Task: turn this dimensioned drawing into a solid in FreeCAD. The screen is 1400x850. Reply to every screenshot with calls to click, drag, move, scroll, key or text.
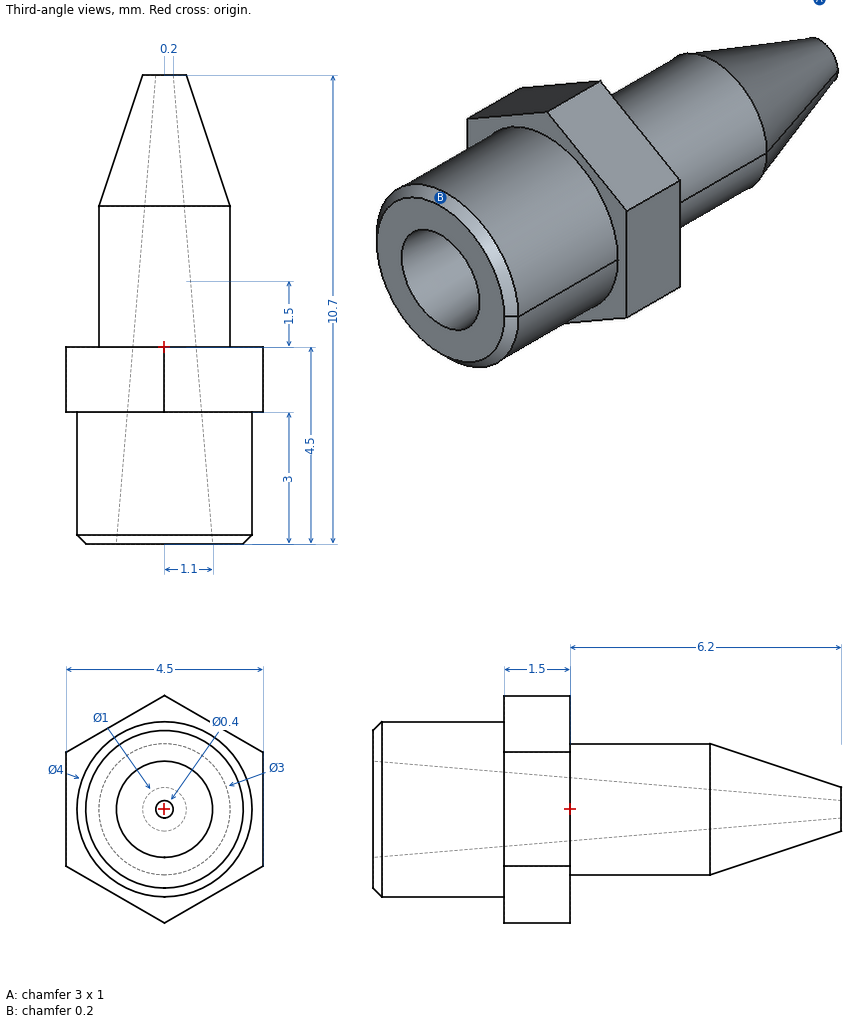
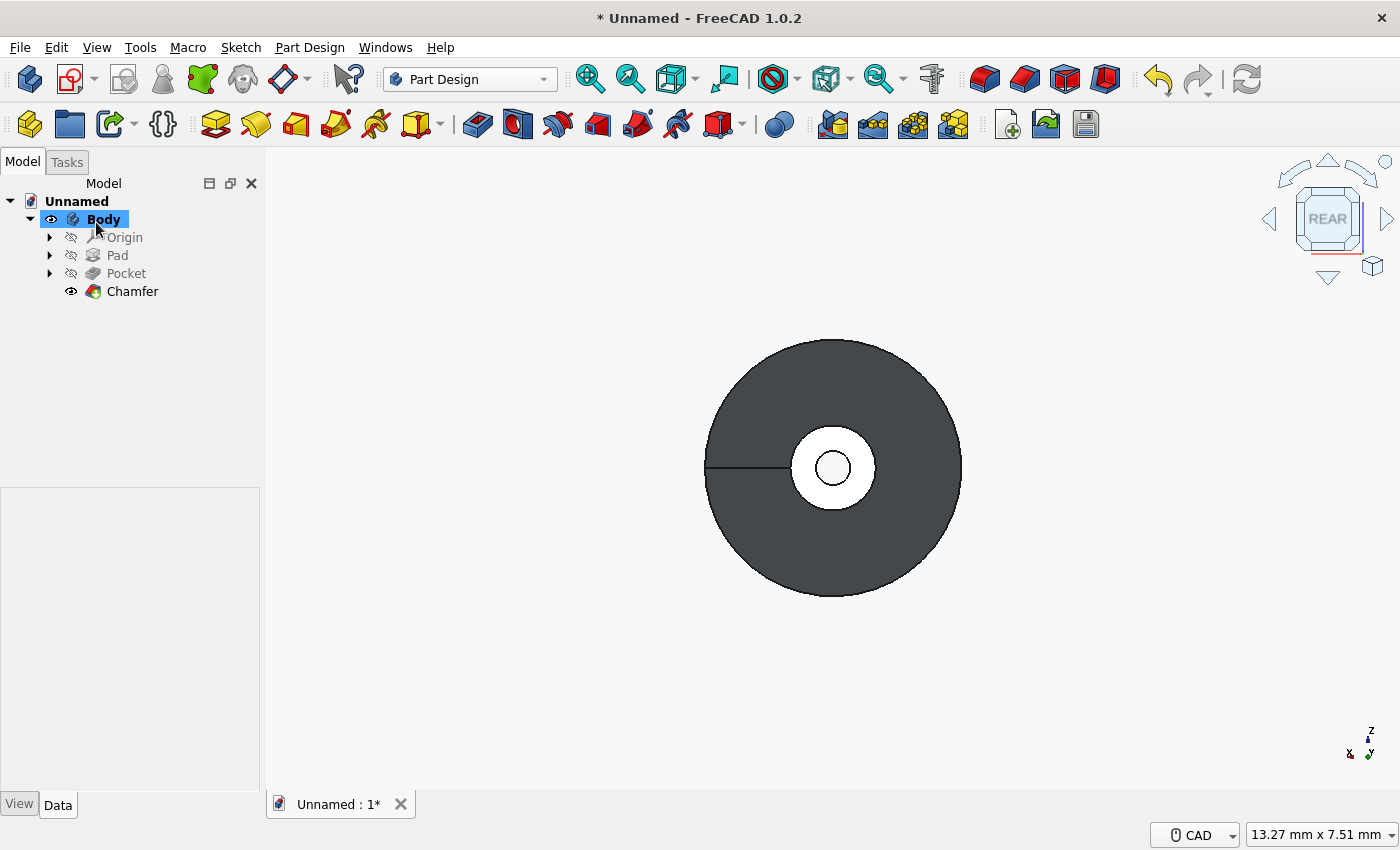
click(592, 80)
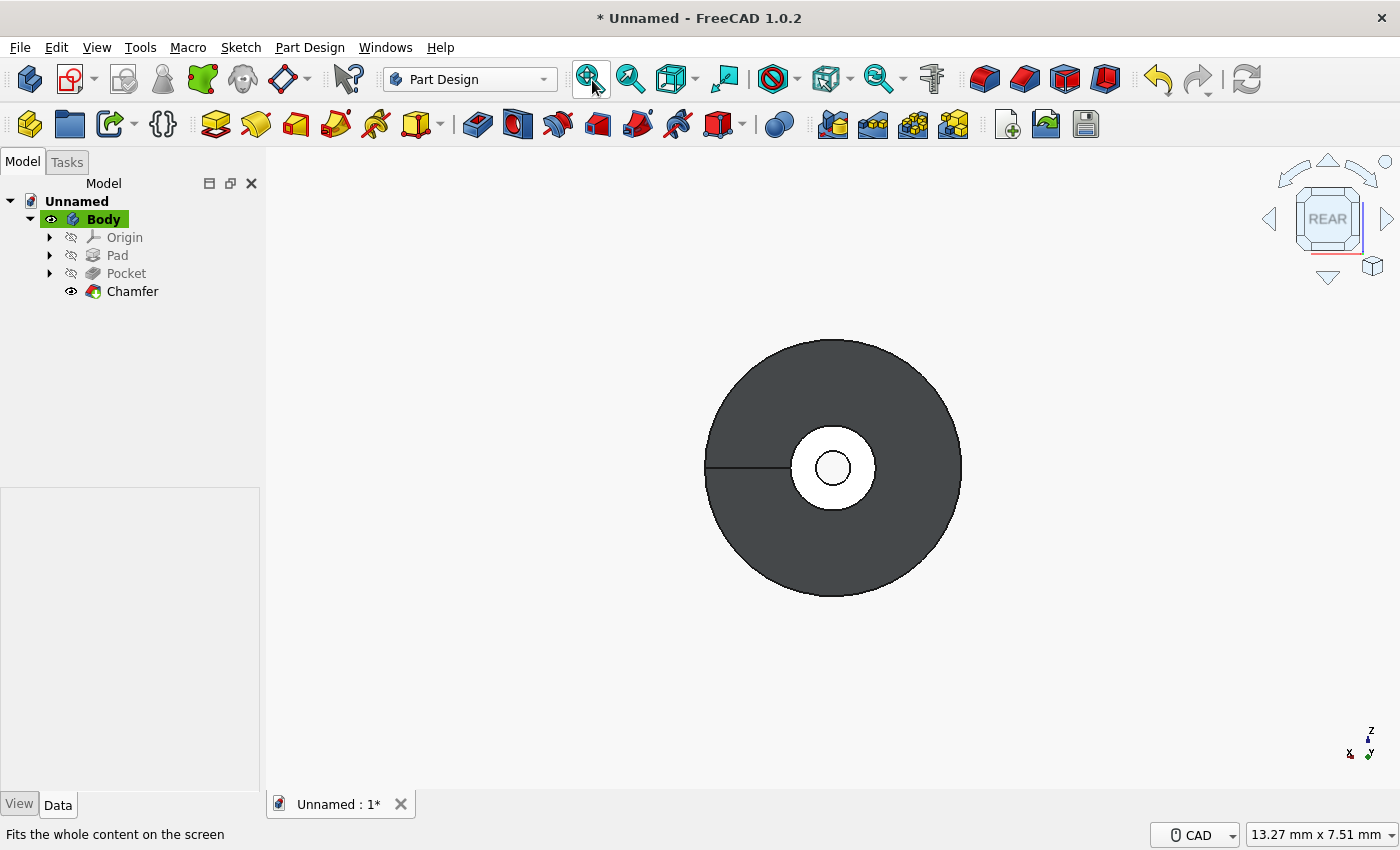
click(70, 80)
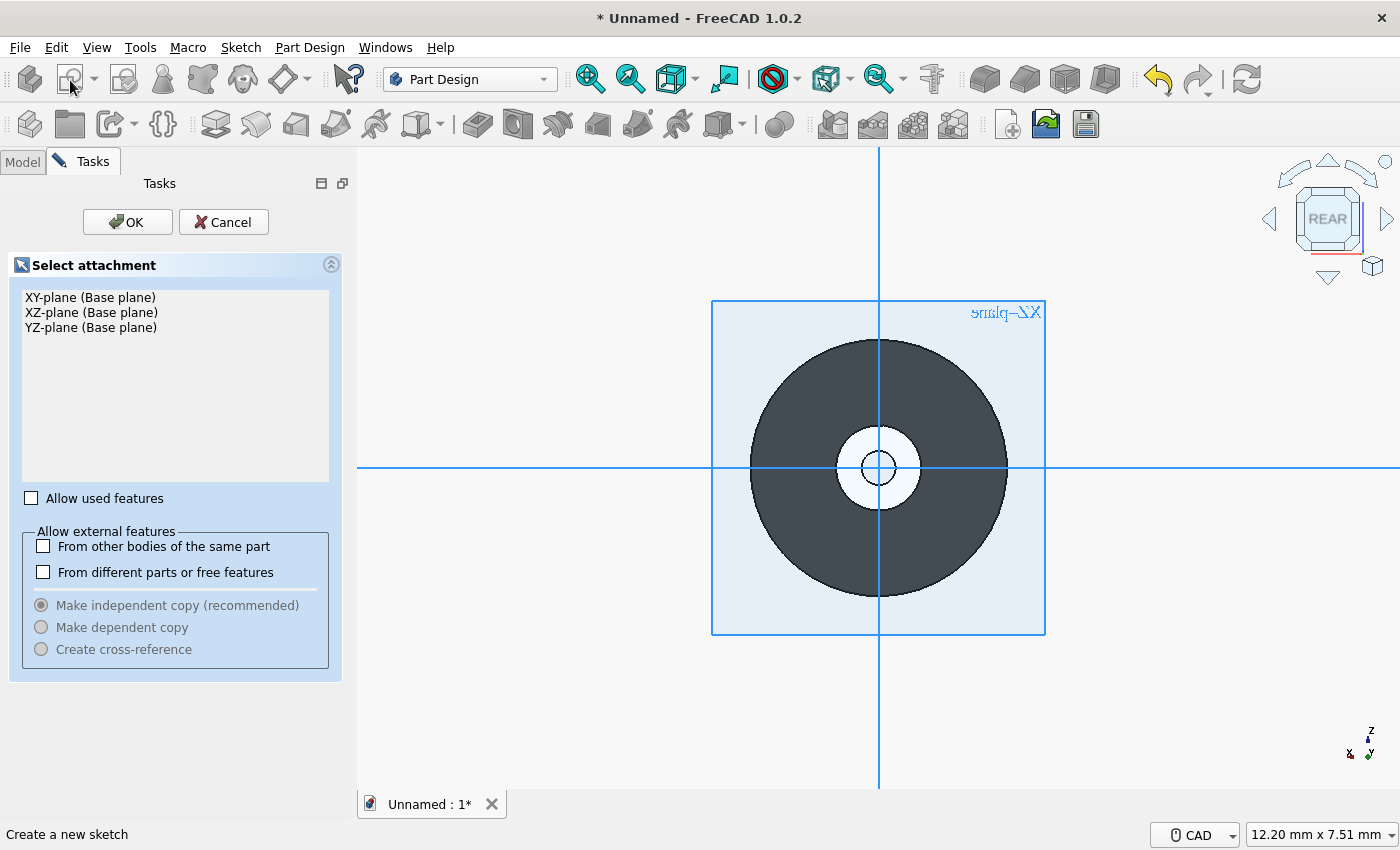
click(82, 312)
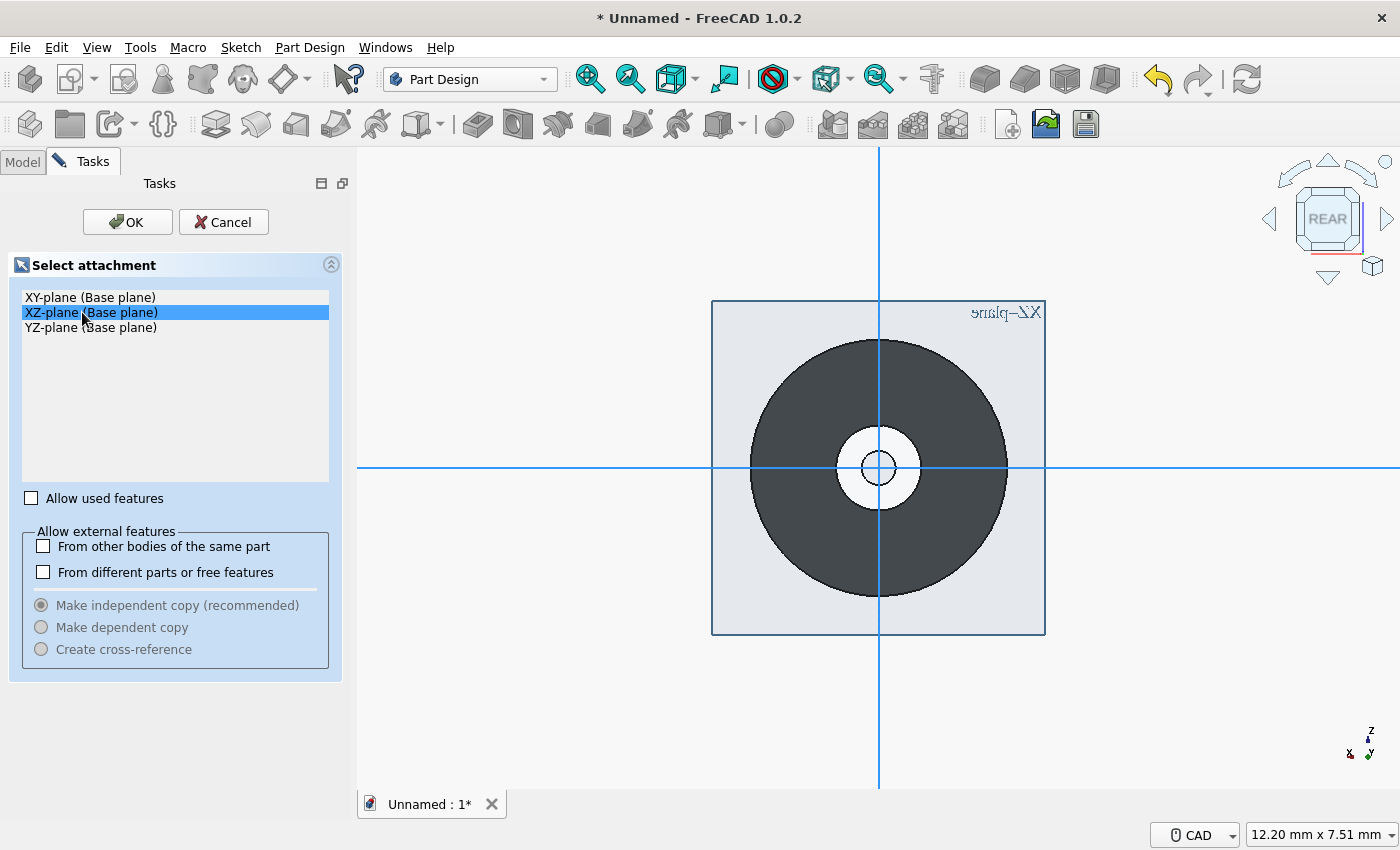
click(128, 222)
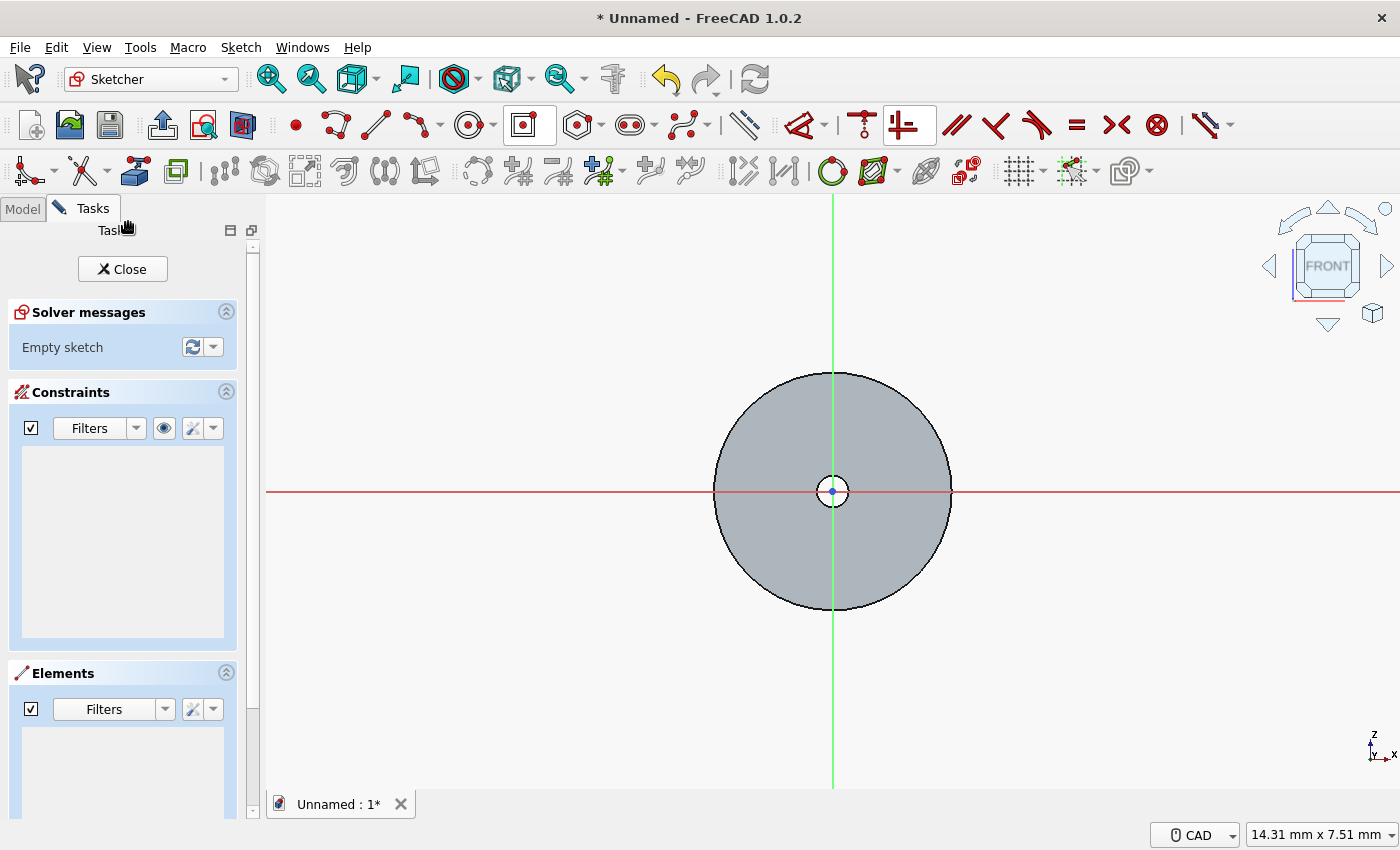
scroll(850, 492, up, 8)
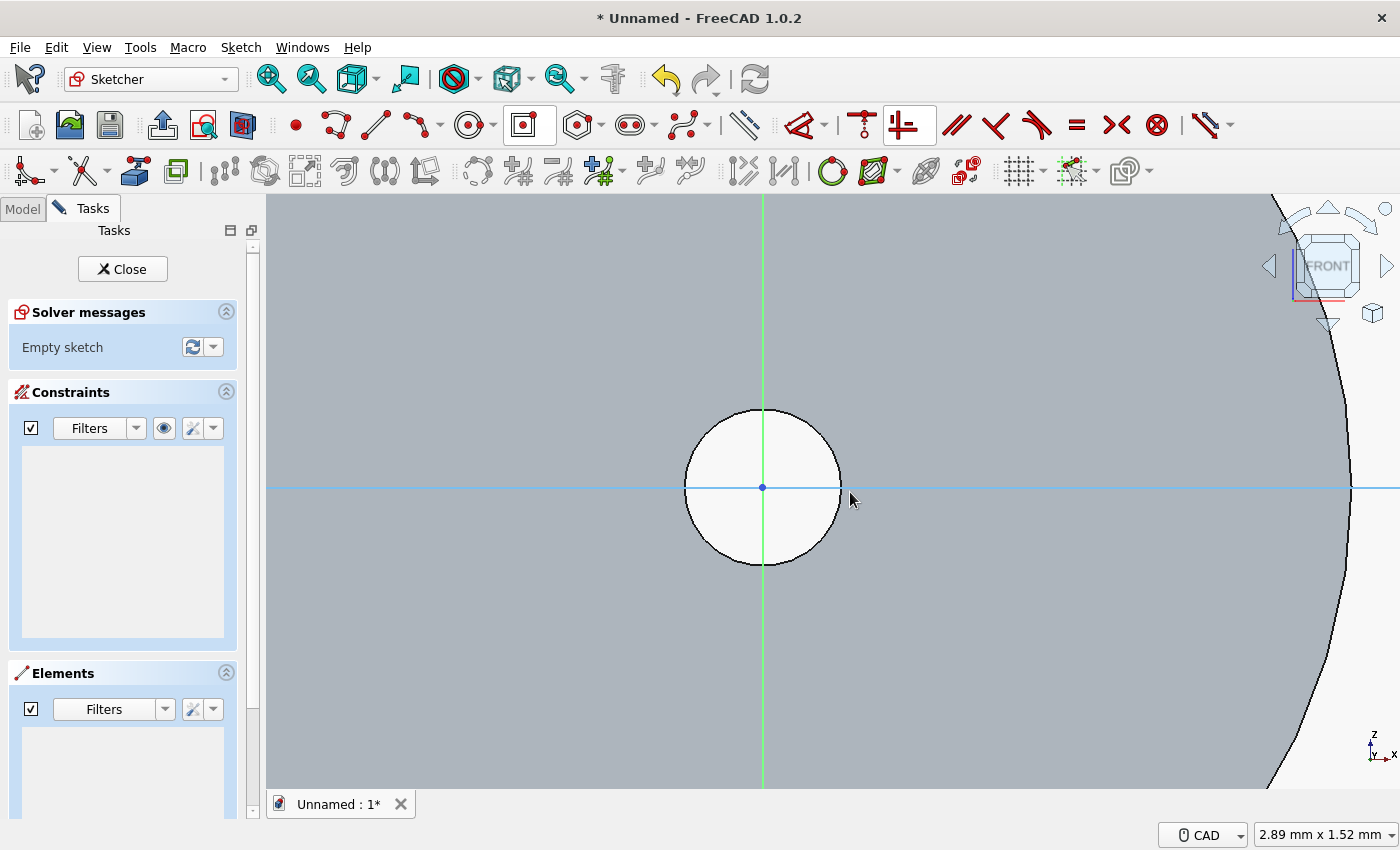
click(470, 126)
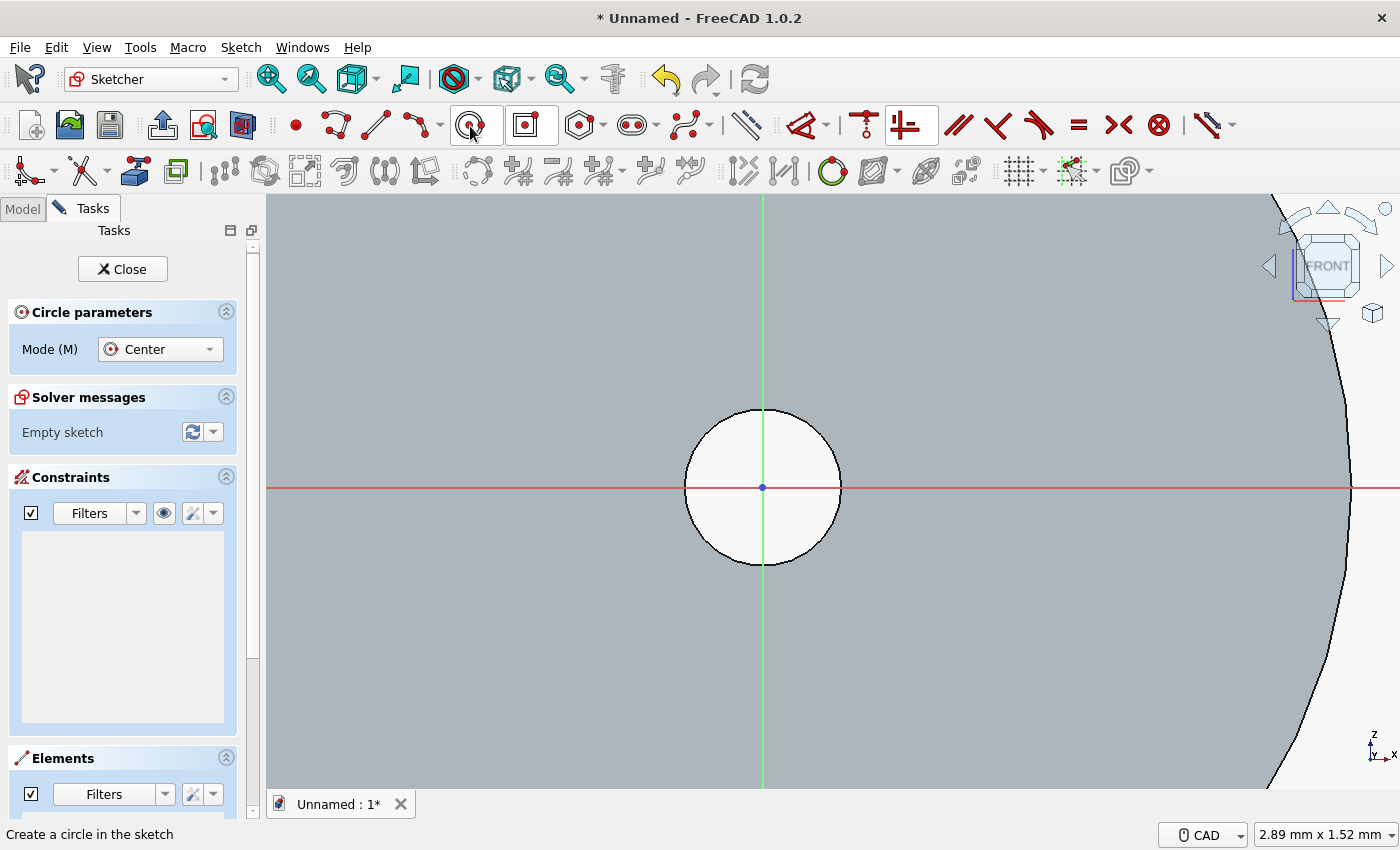
click(763, 488)
click(902, 349)
key(Escape)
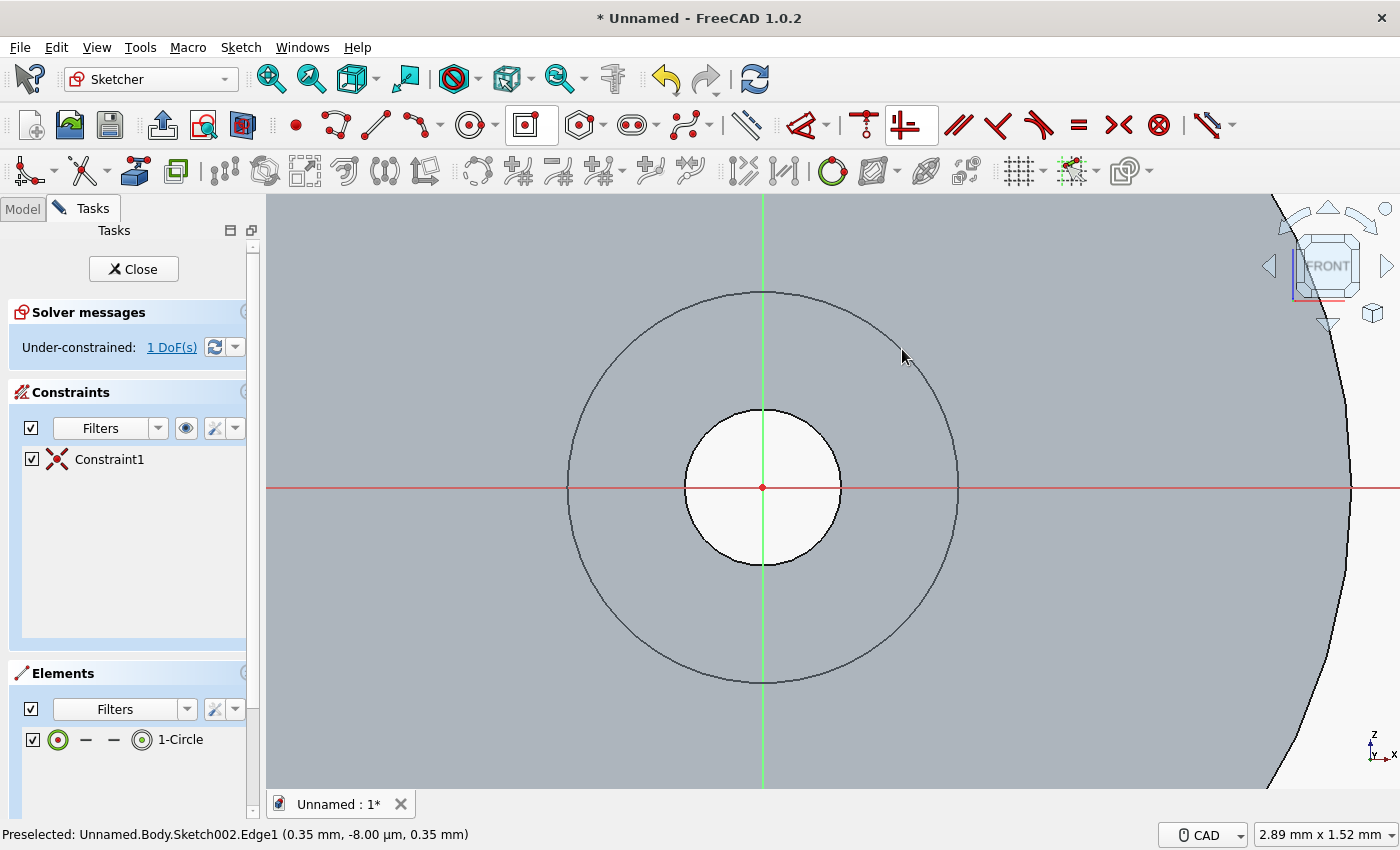
click(901, 349)